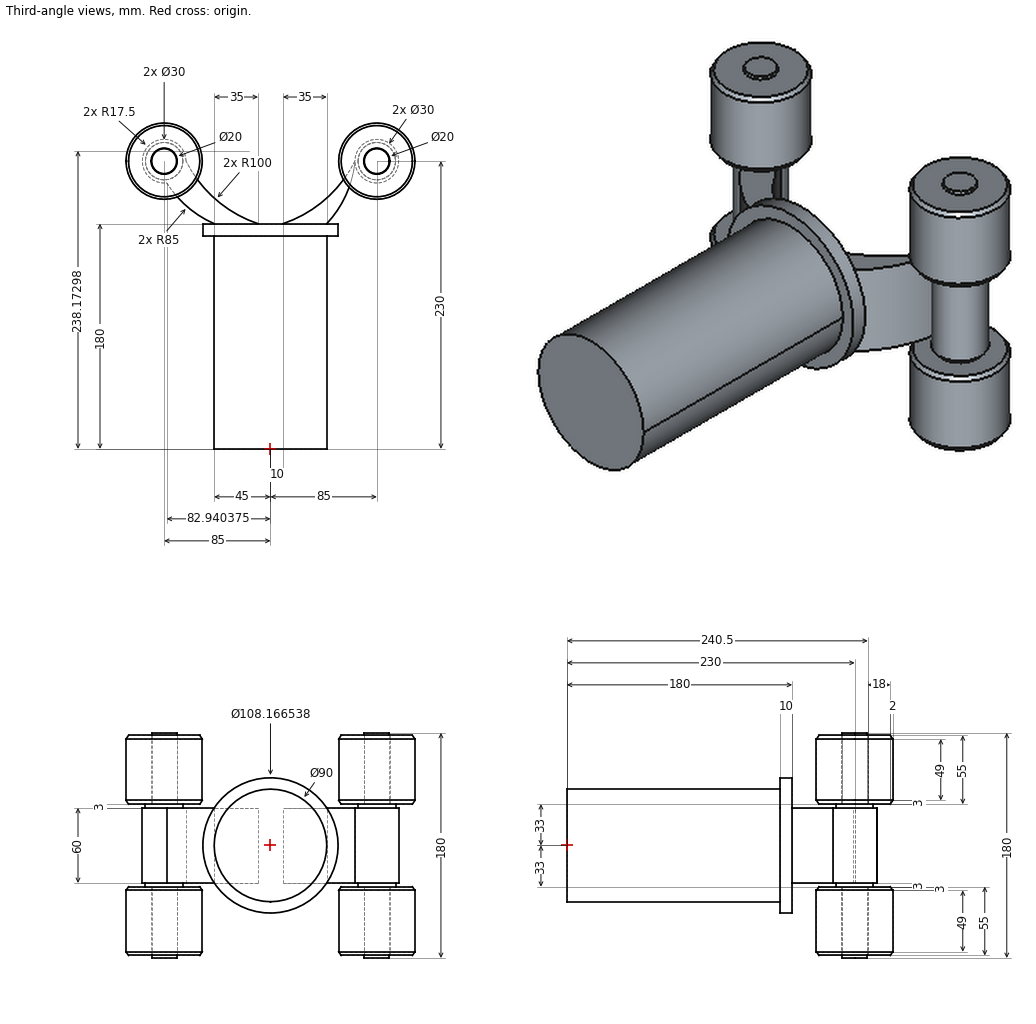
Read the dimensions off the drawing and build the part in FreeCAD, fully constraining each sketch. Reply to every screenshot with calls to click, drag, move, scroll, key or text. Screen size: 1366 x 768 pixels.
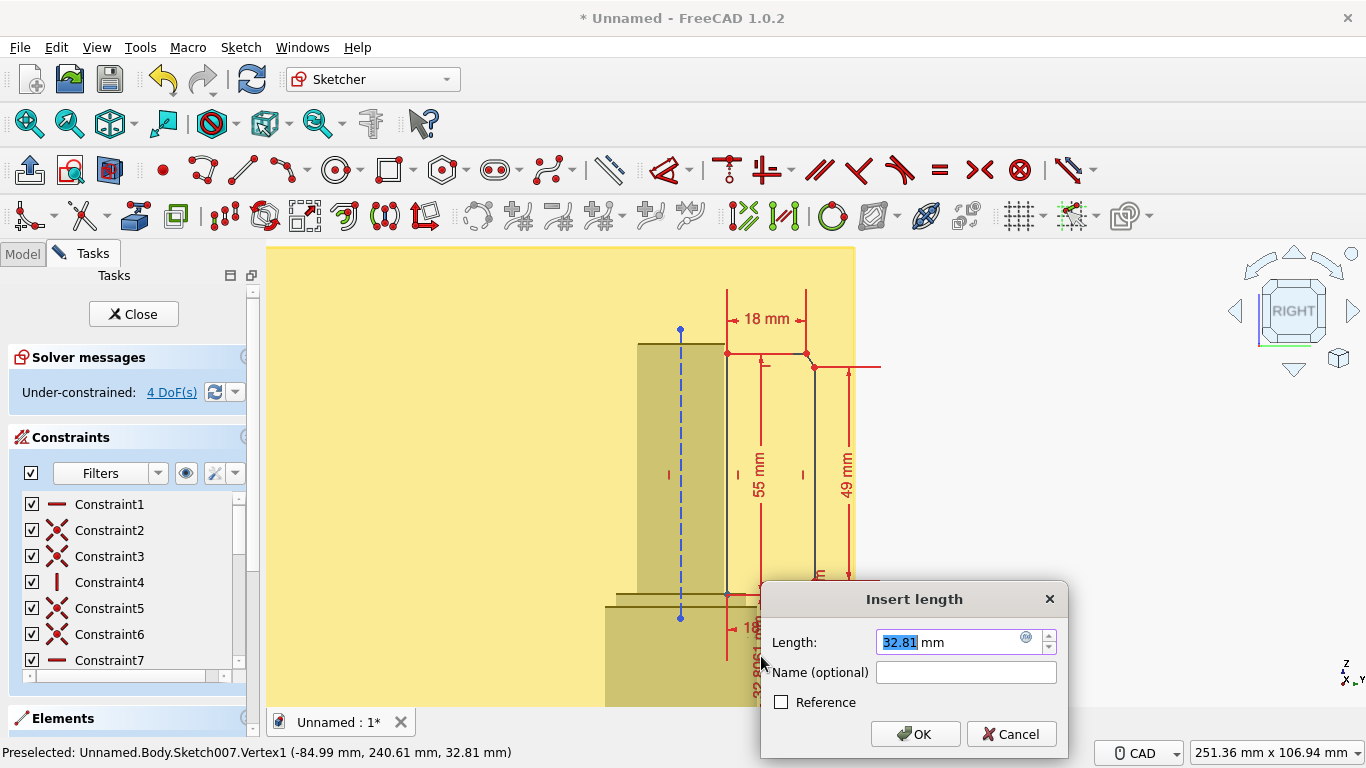
text(33)
key(Return)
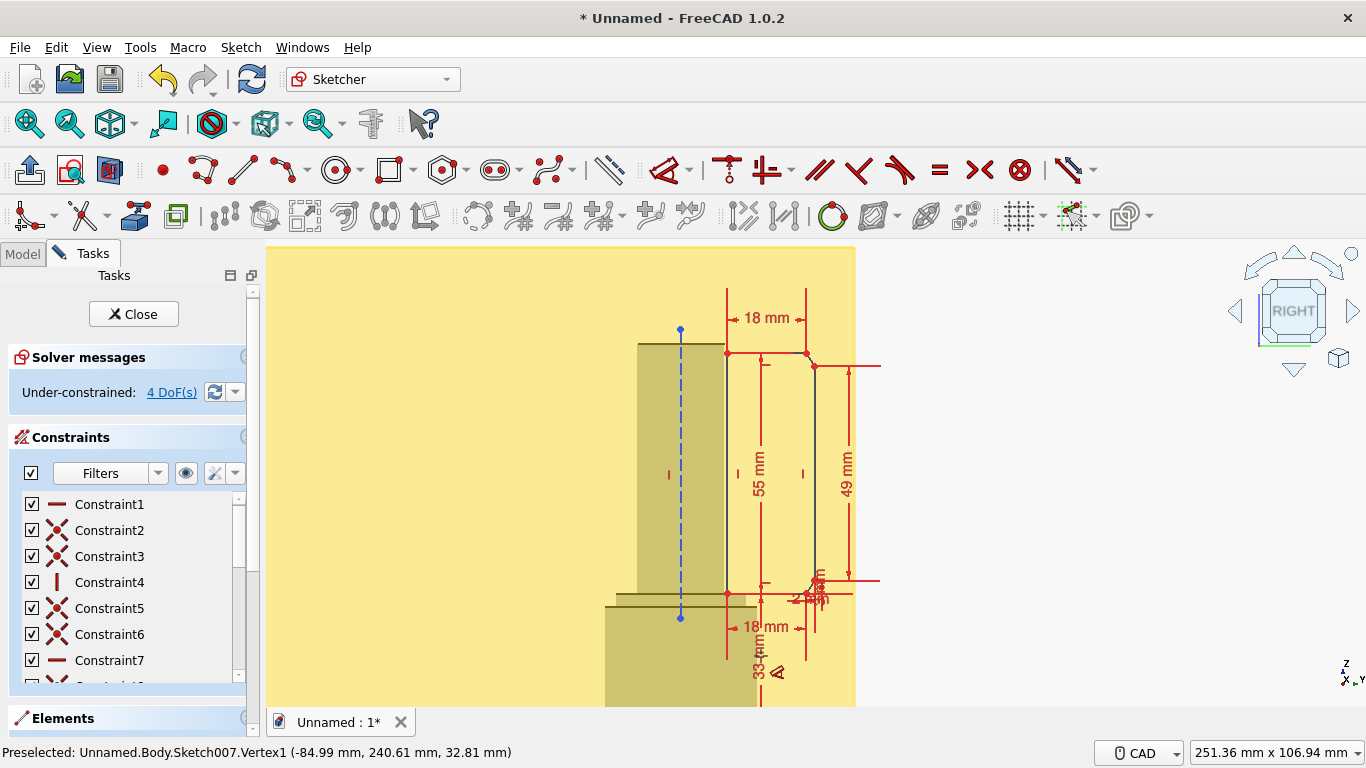
click(681, 619)
click(487, 585)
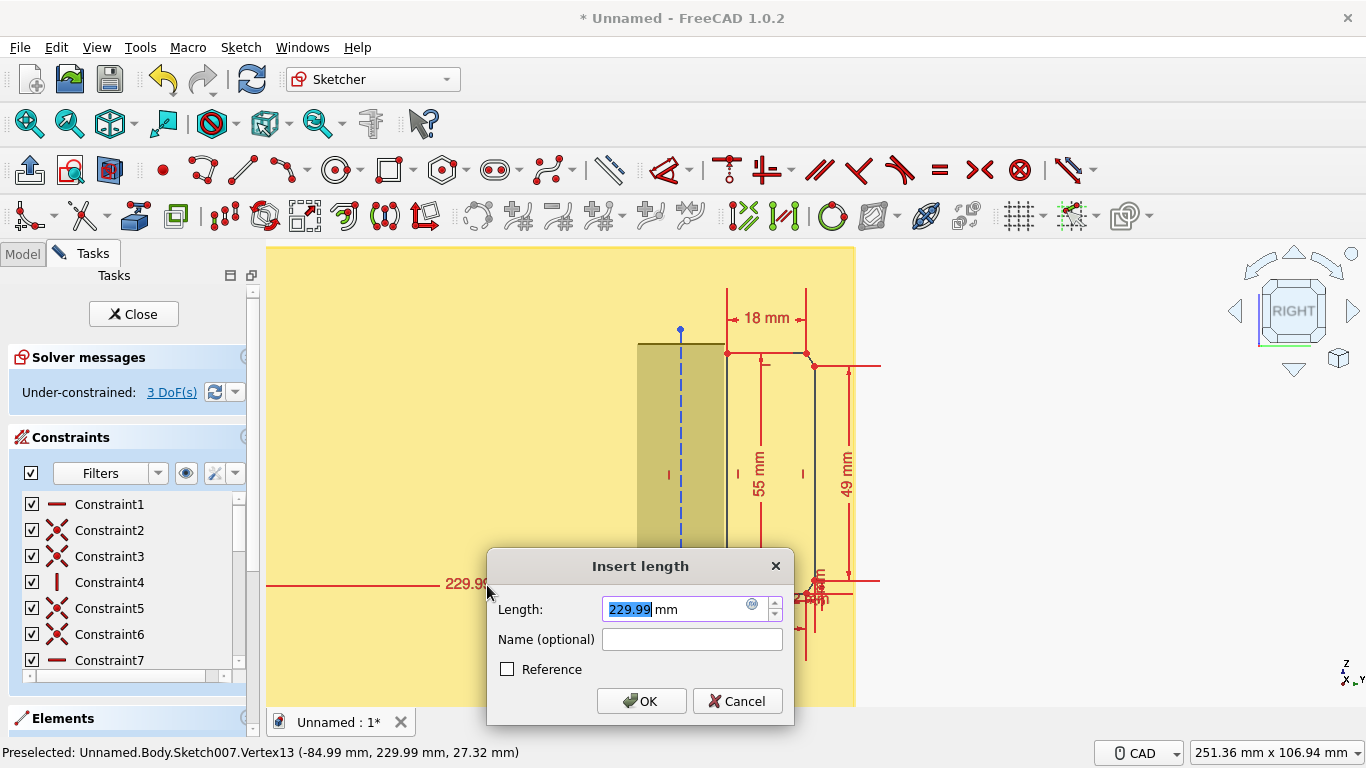
text(230)
key(Return)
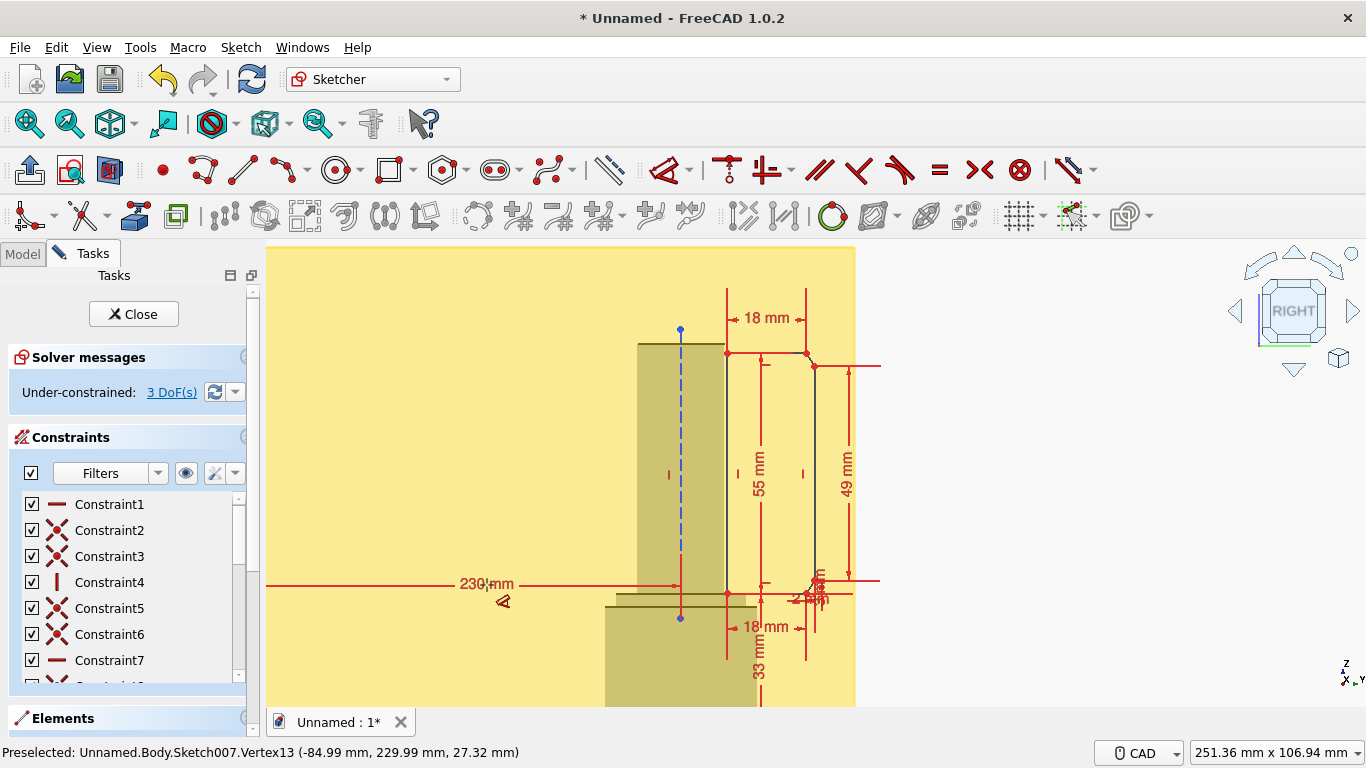
click(727, 594)
click(511, 560)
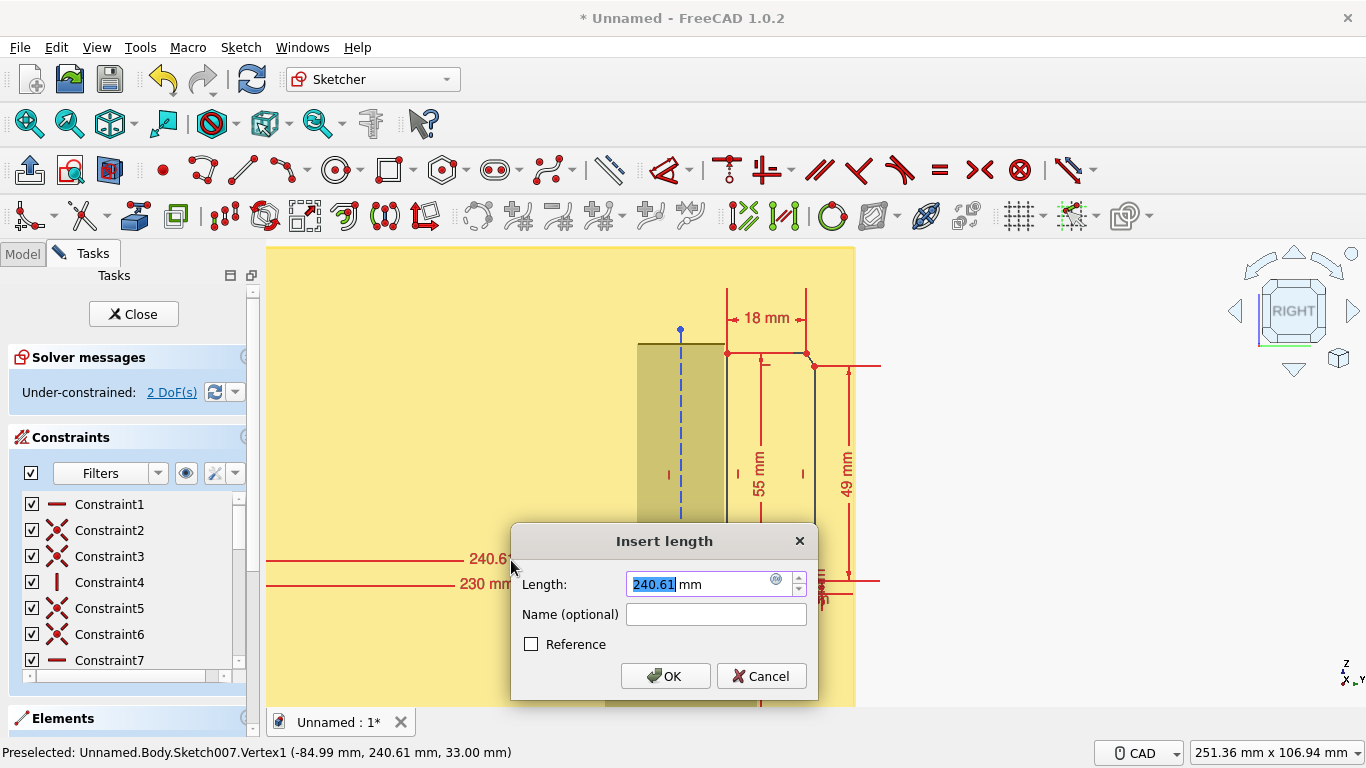
text(240.5)
key(Return)
key(Escape)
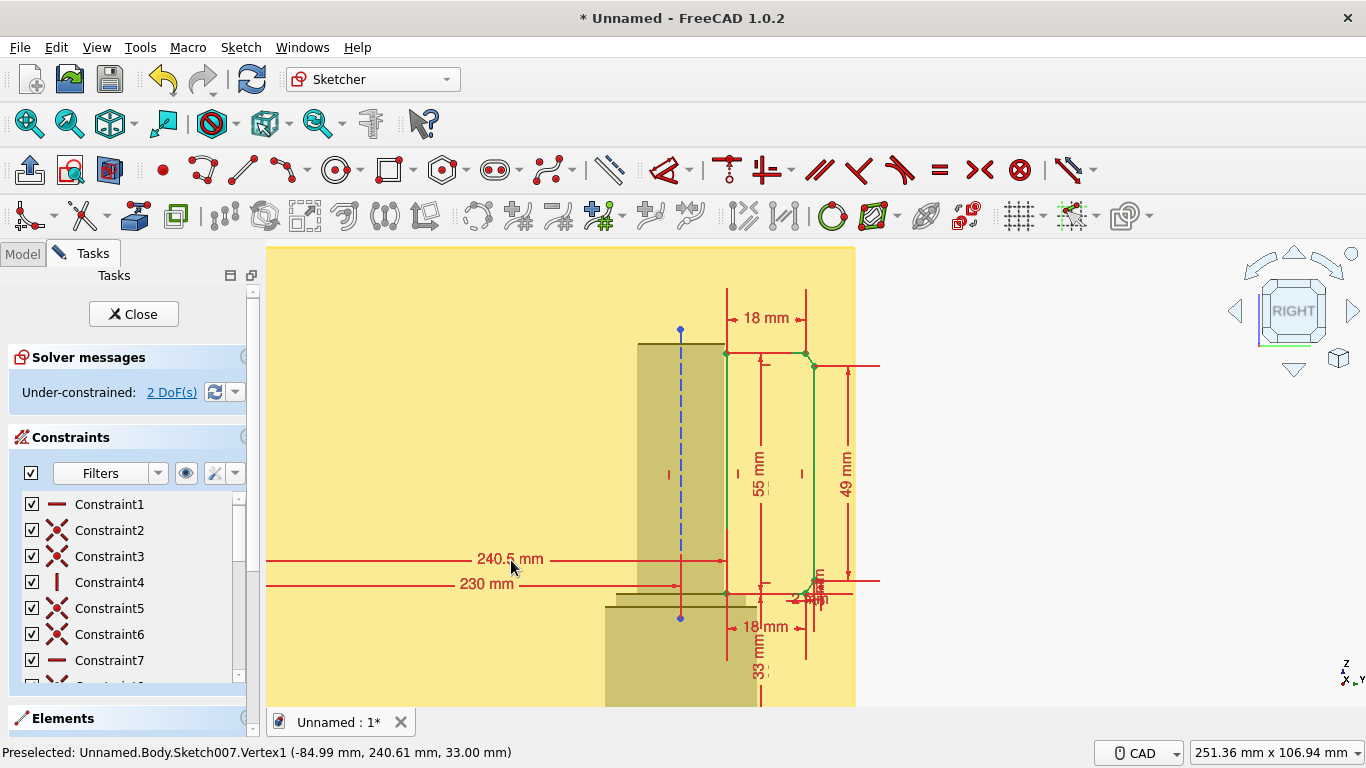
click(134, 314)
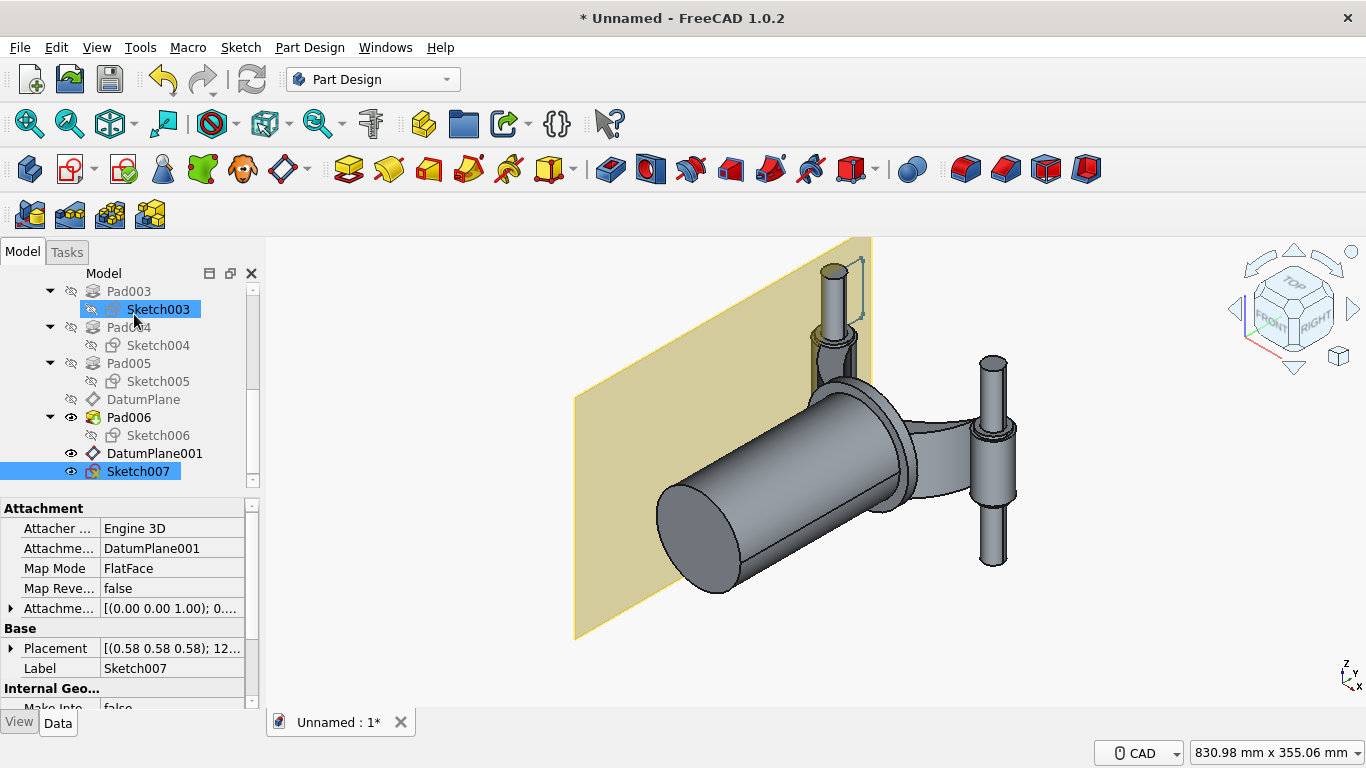
click(390, 170)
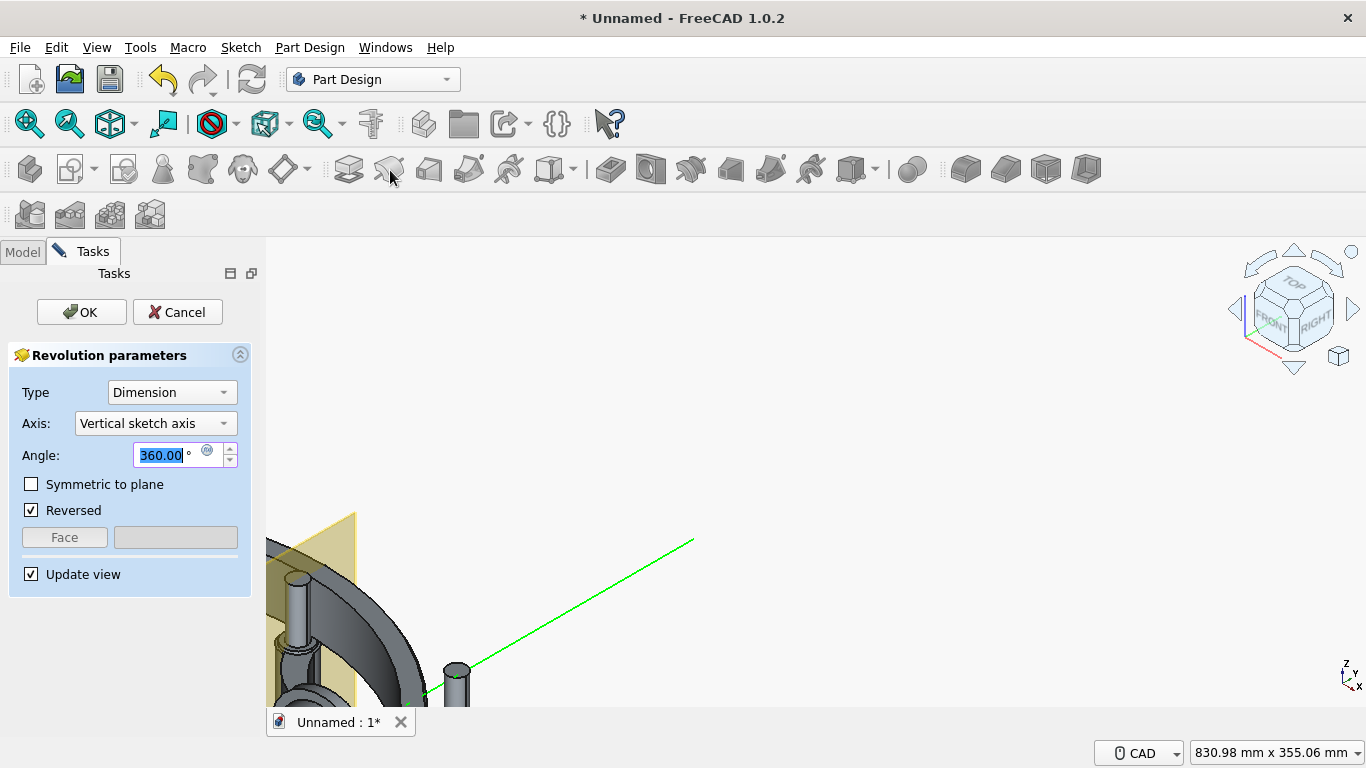
click(156, 424)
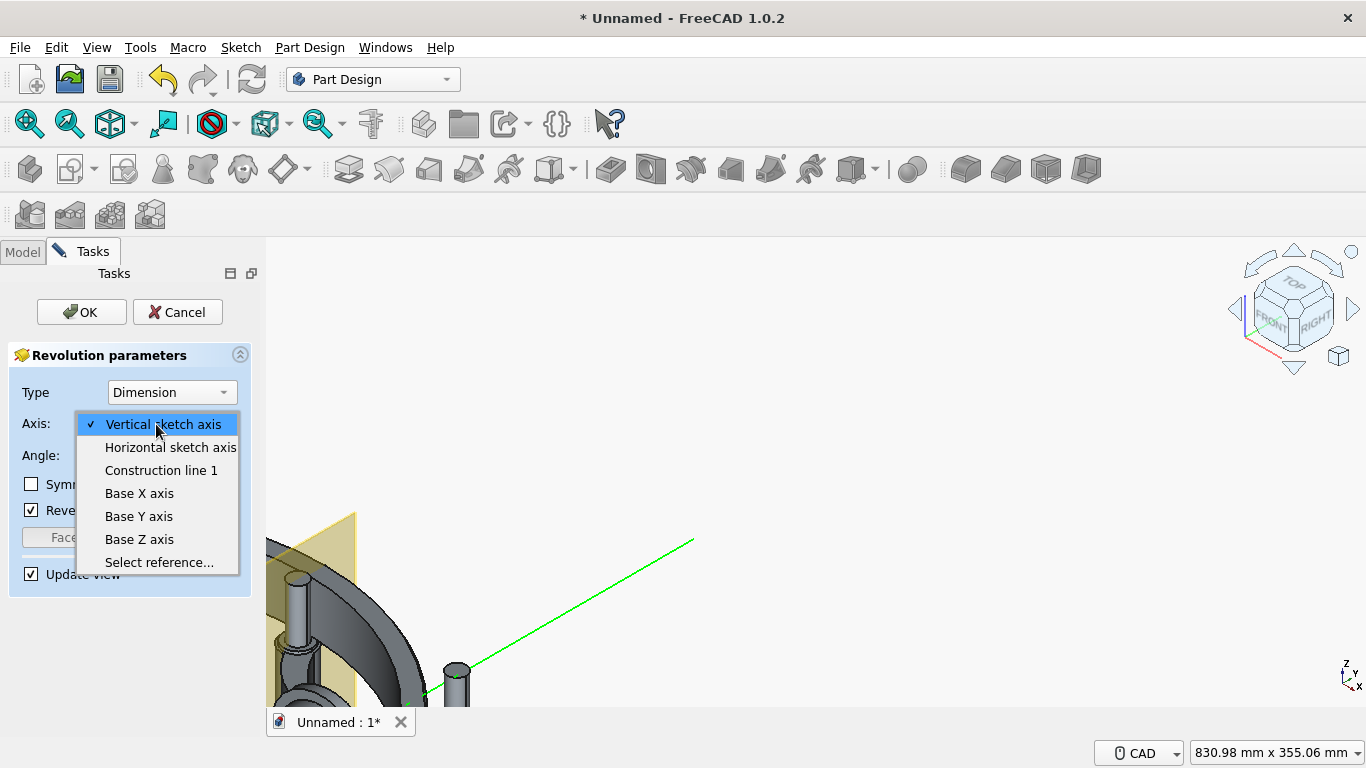
click(156, 470)